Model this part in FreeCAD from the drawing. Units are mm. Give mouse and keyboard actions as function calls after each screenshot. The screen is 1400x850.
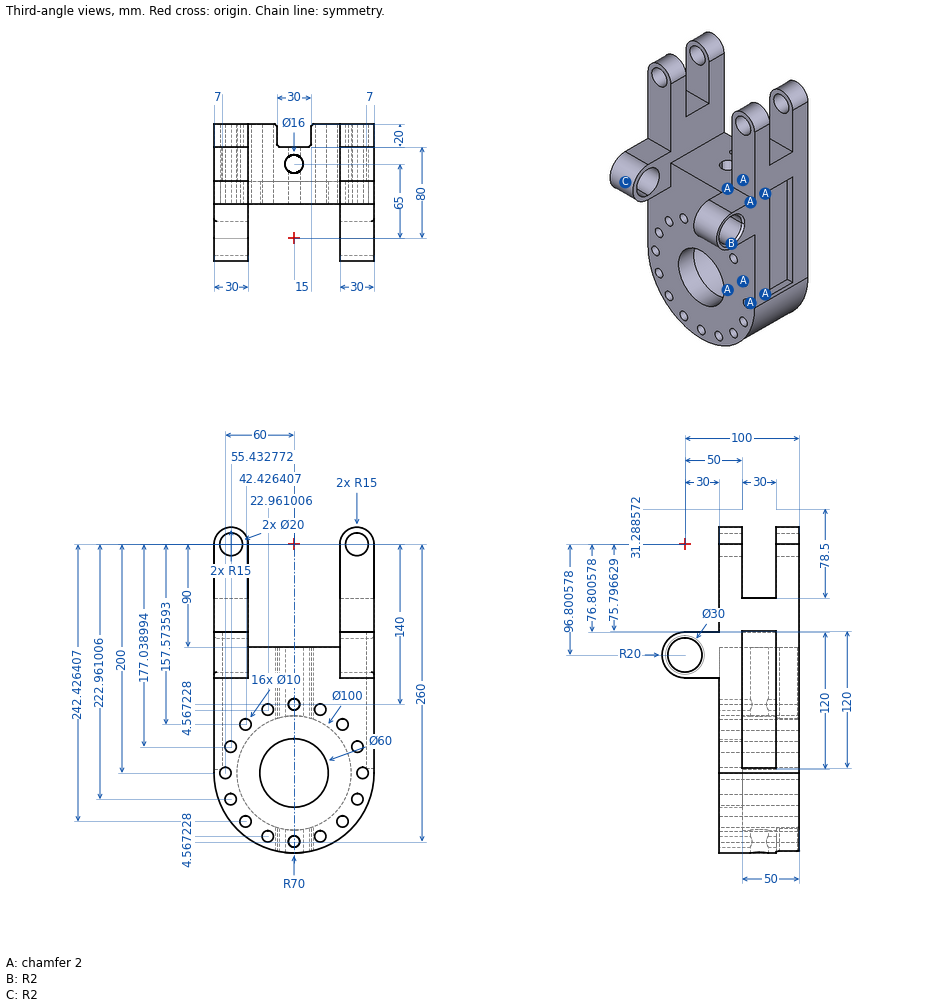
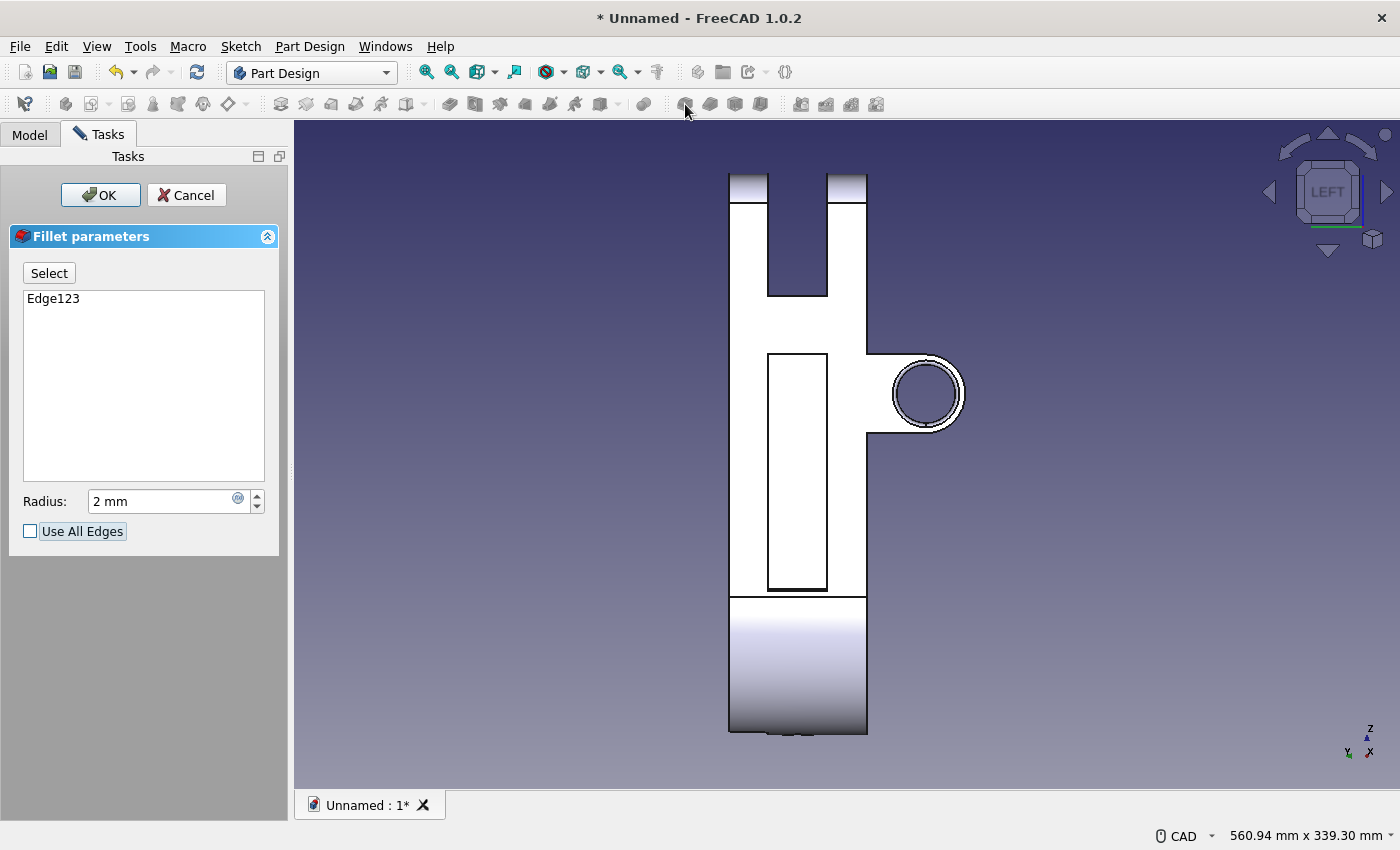
click(101, 195)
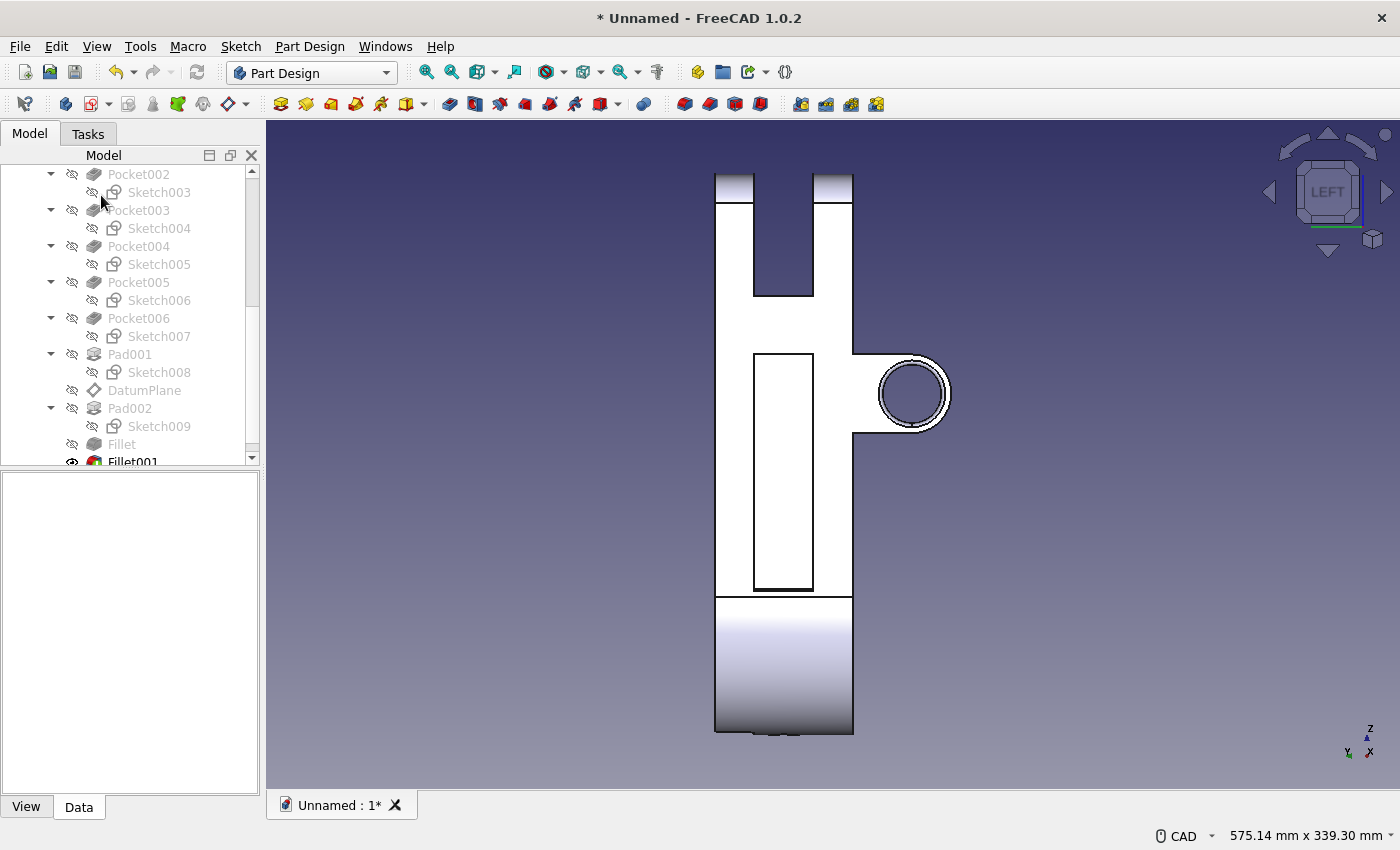
key(0)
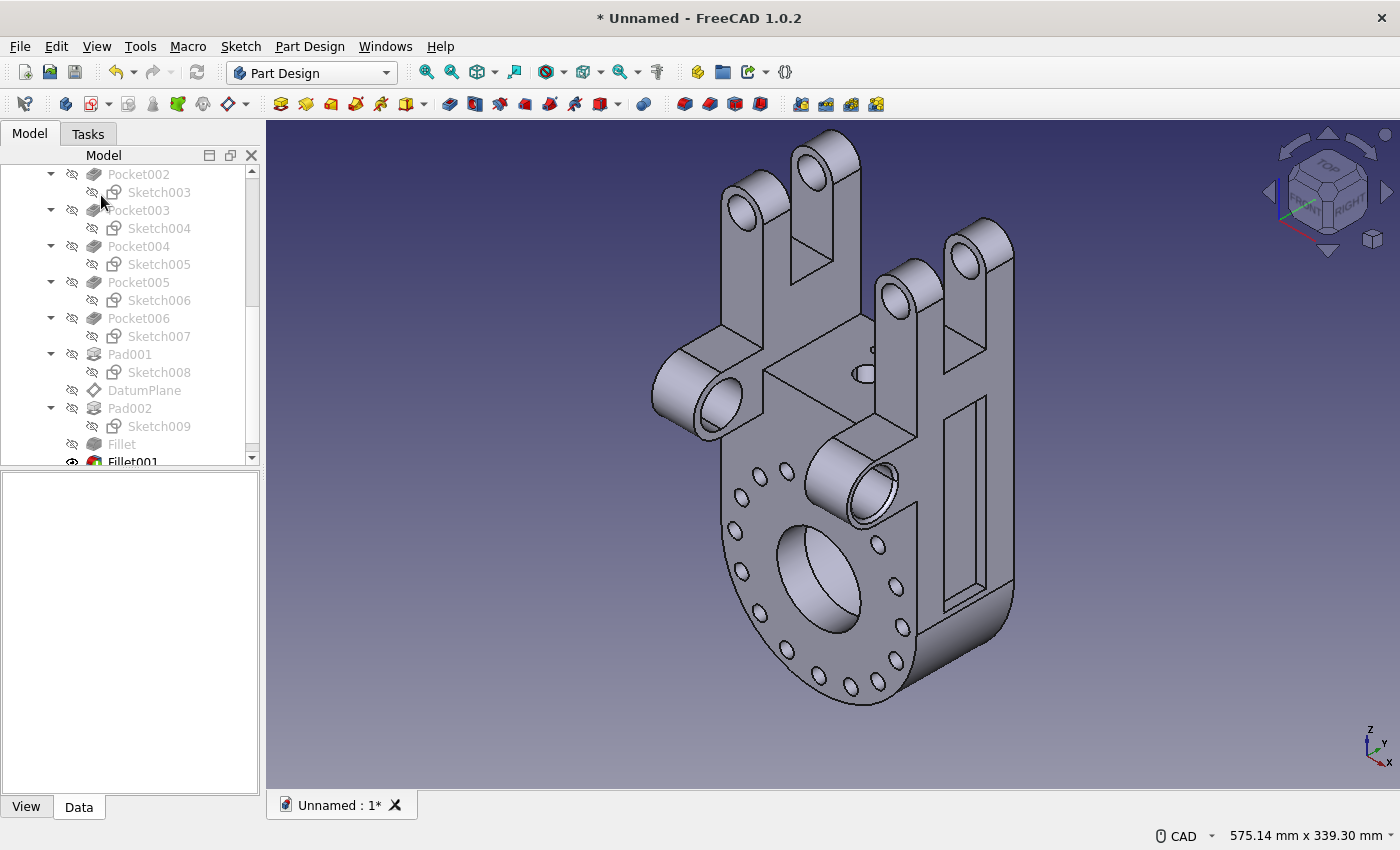
key(v)
key(f)